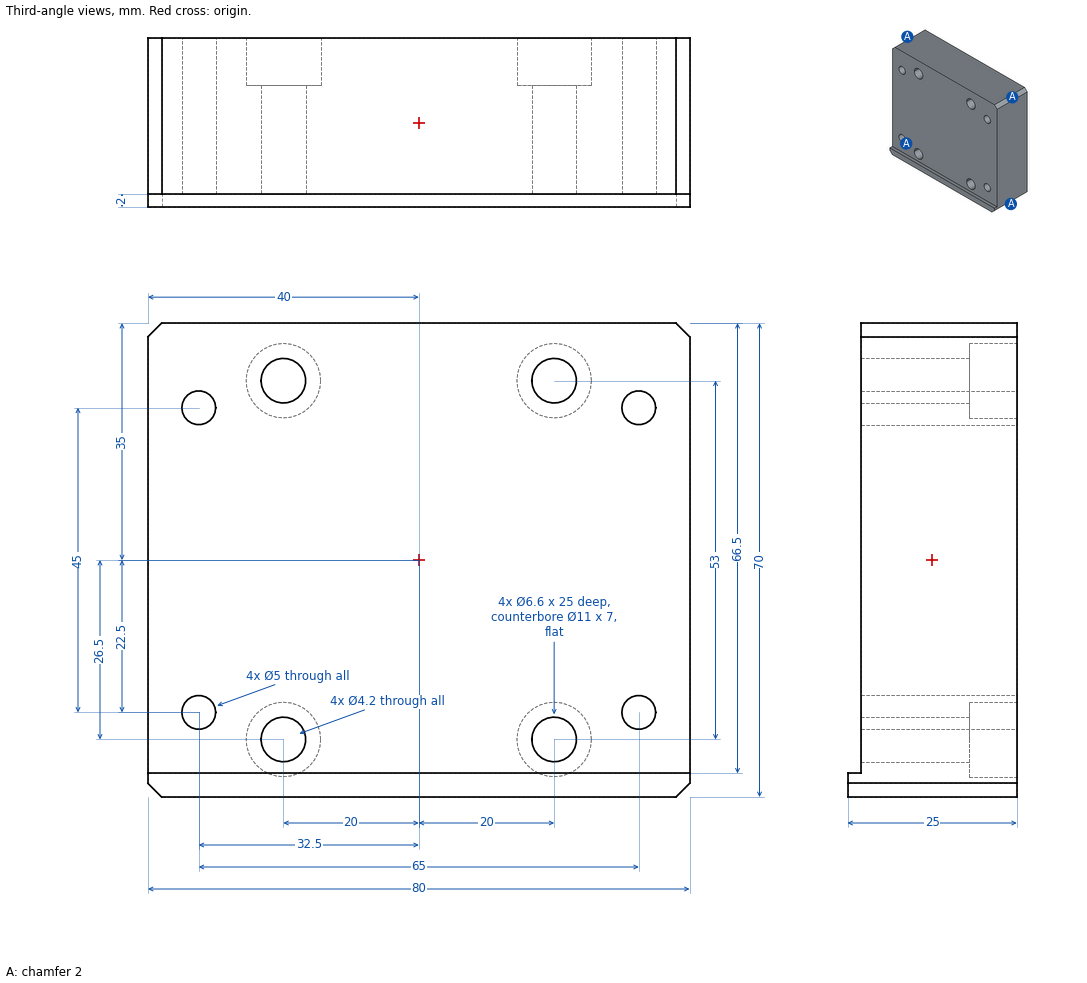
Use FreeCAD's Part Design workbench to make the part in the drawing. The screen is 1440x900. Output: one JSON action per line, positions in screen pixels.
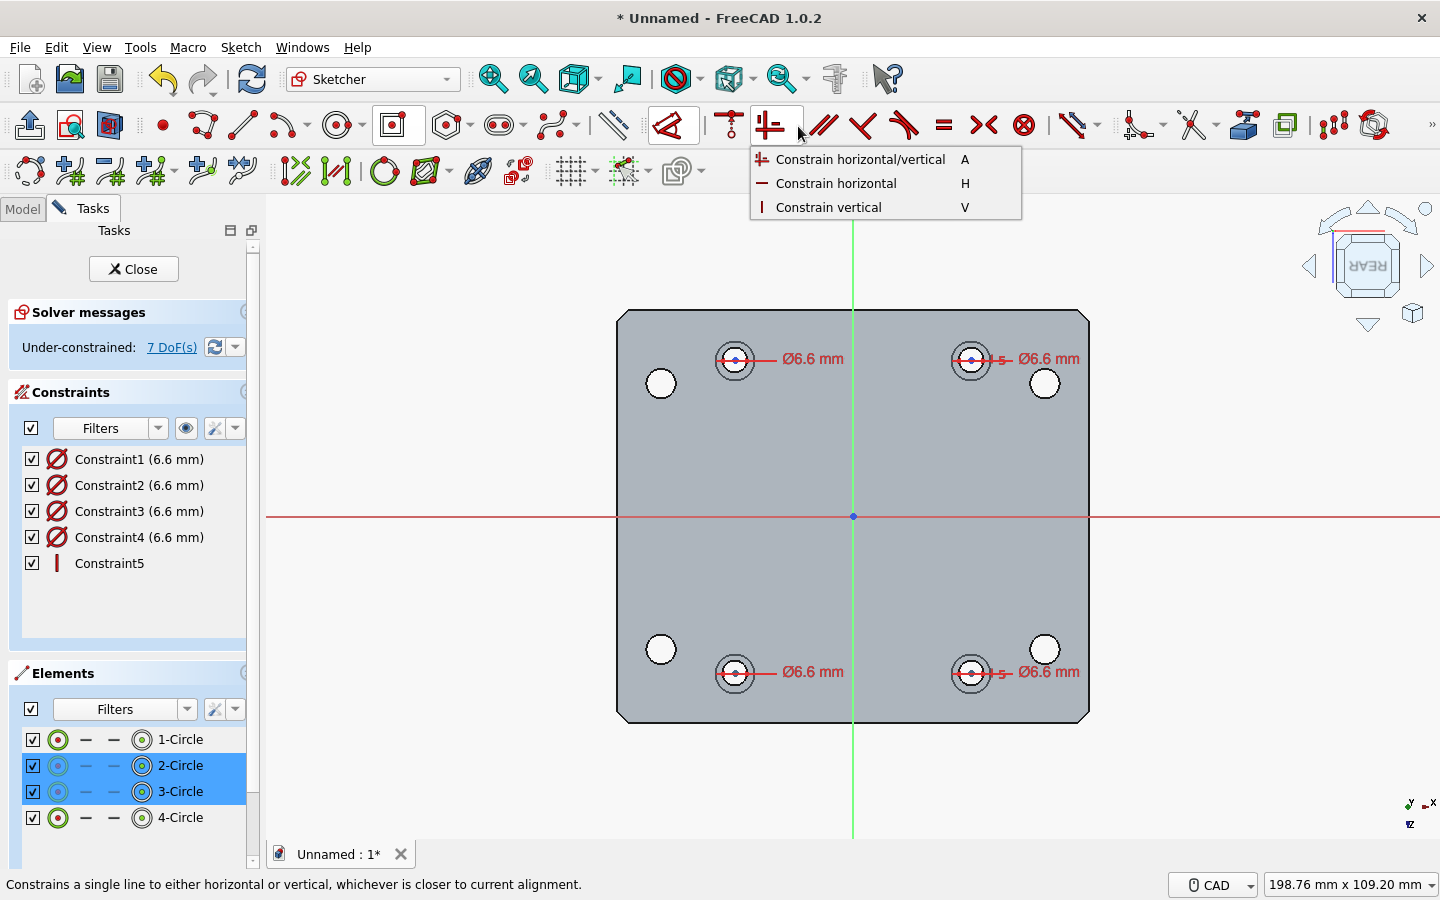
{"action": "left_click", "coordinate": [886, 183]}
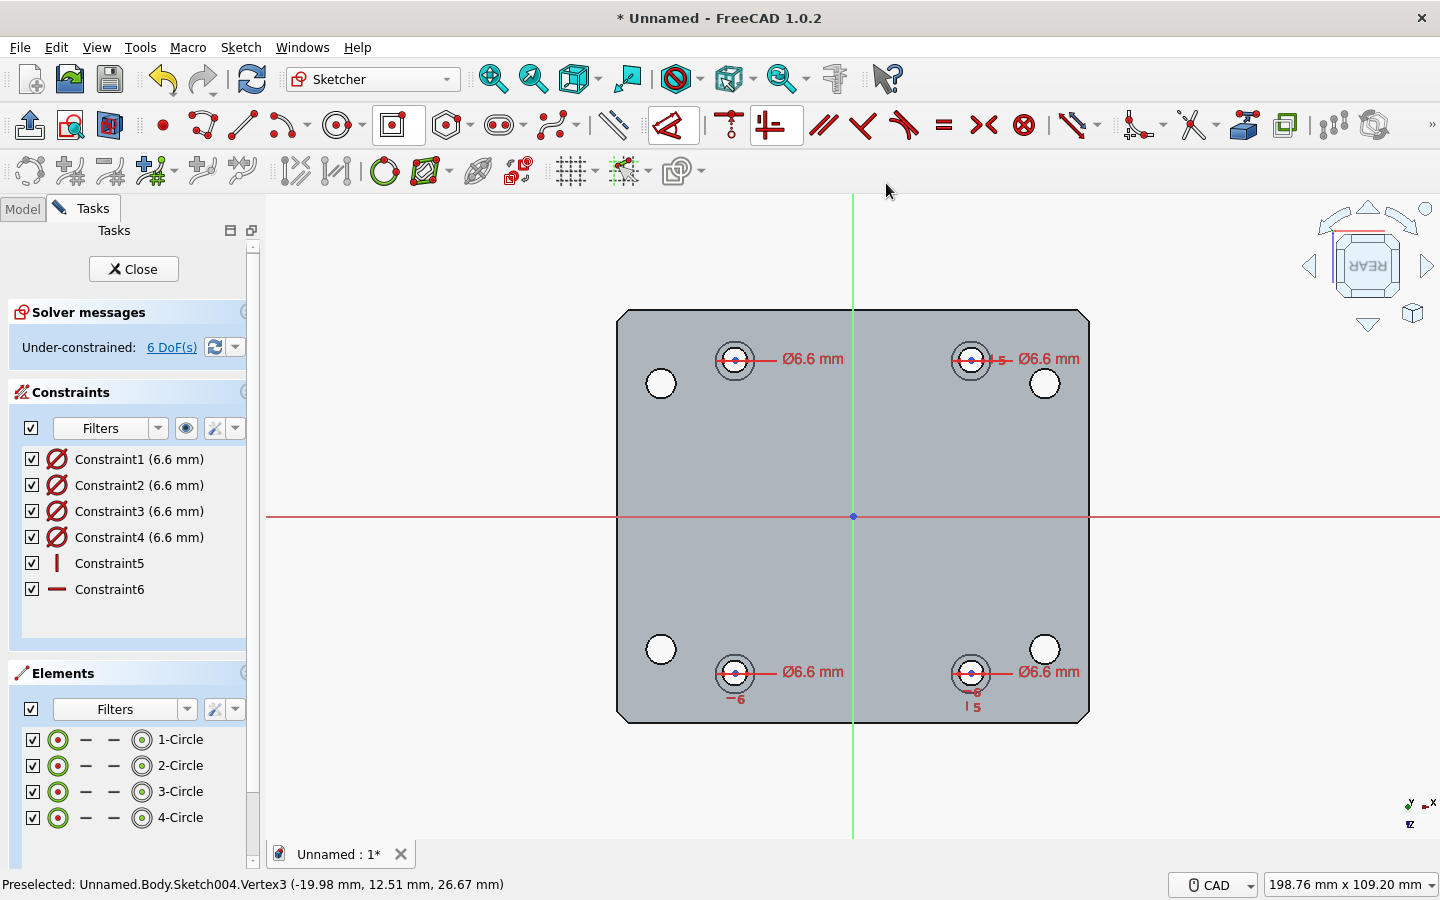
{"action": "left_click", "coordinate": [735, 674]}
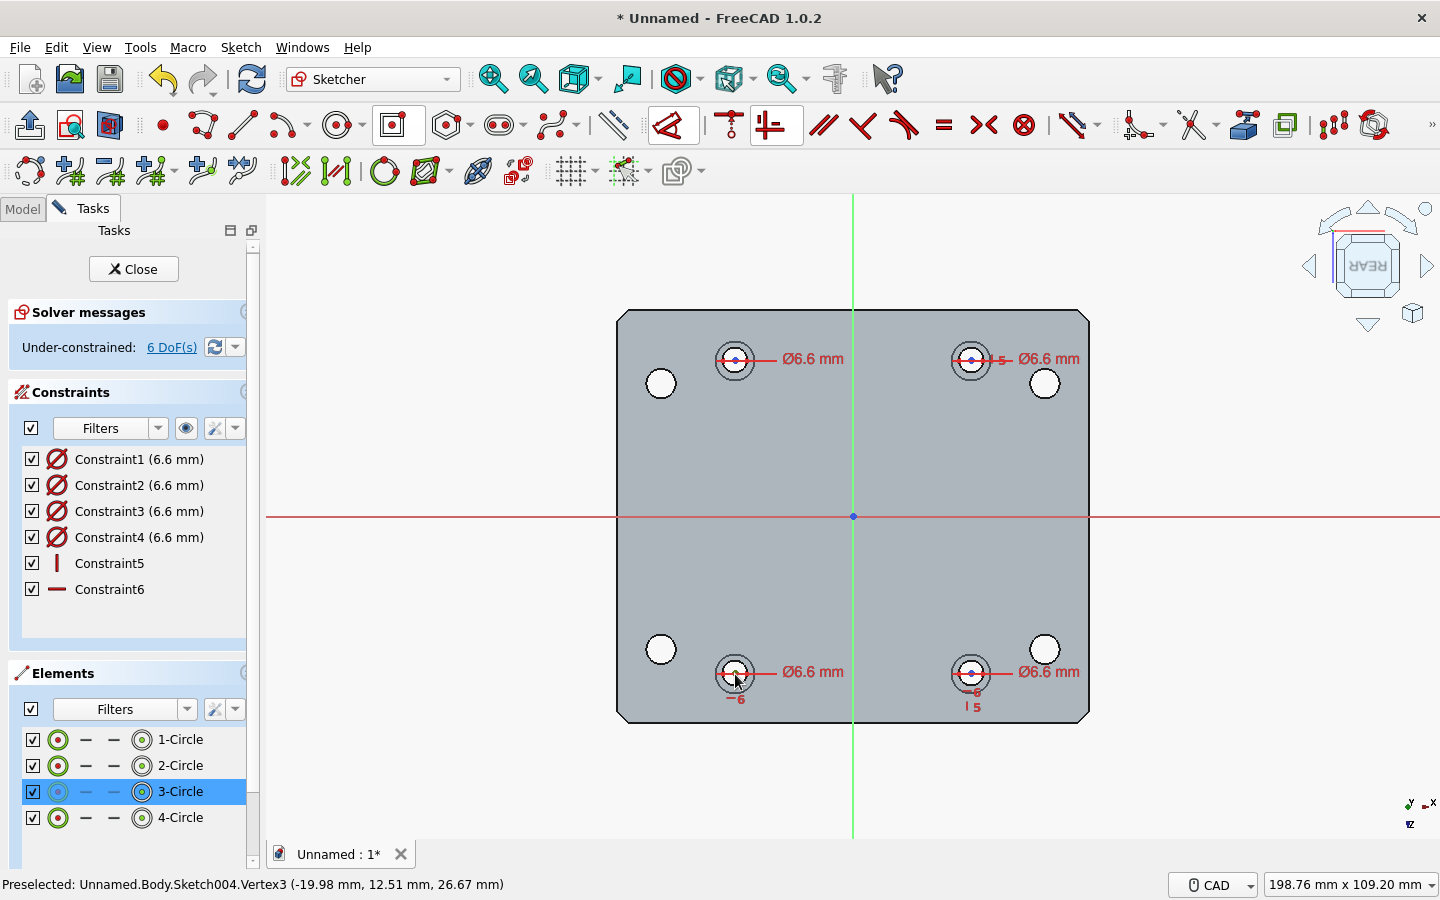
{"action": "left_click", "coordinate": [735, 361]}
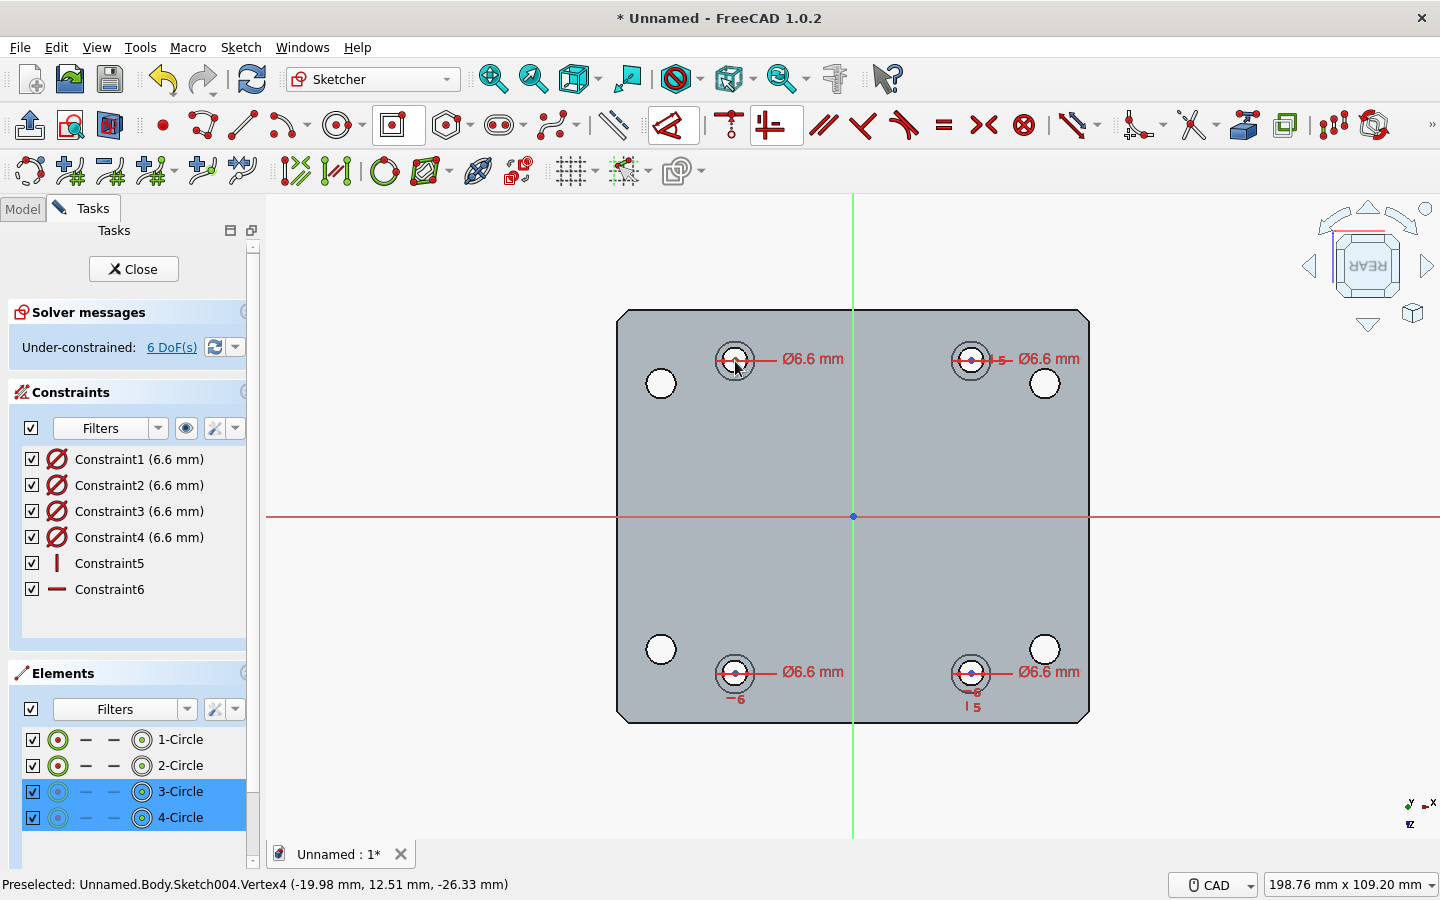
{"action": "left_click", "coordinate": [798, 126]}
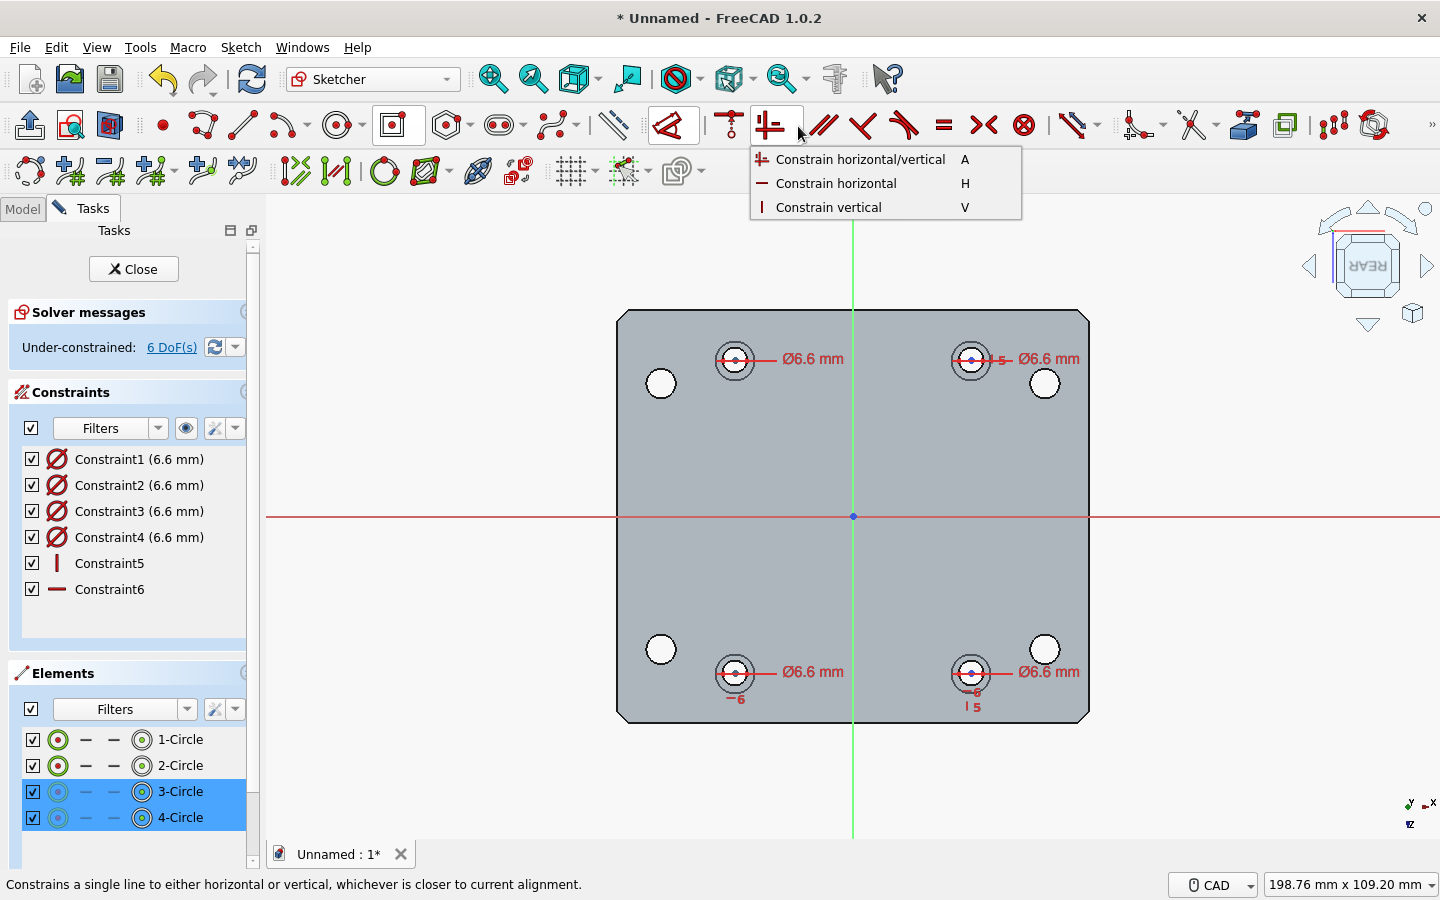
{"action": "left_click", "coordinate": [886, 207]}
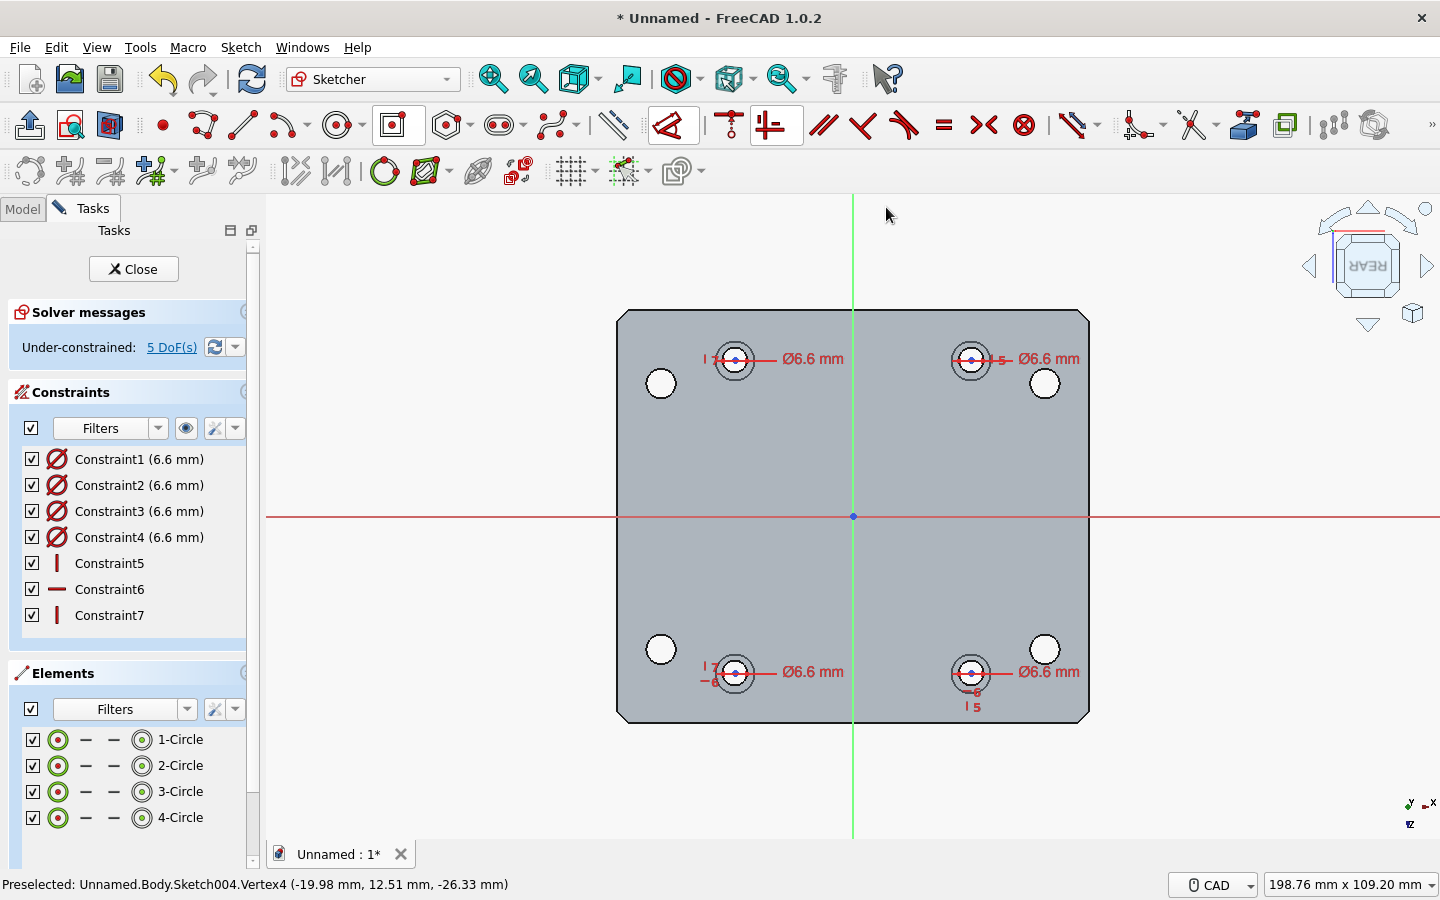
{"action": "left_click", "coordinate": [971, 361]}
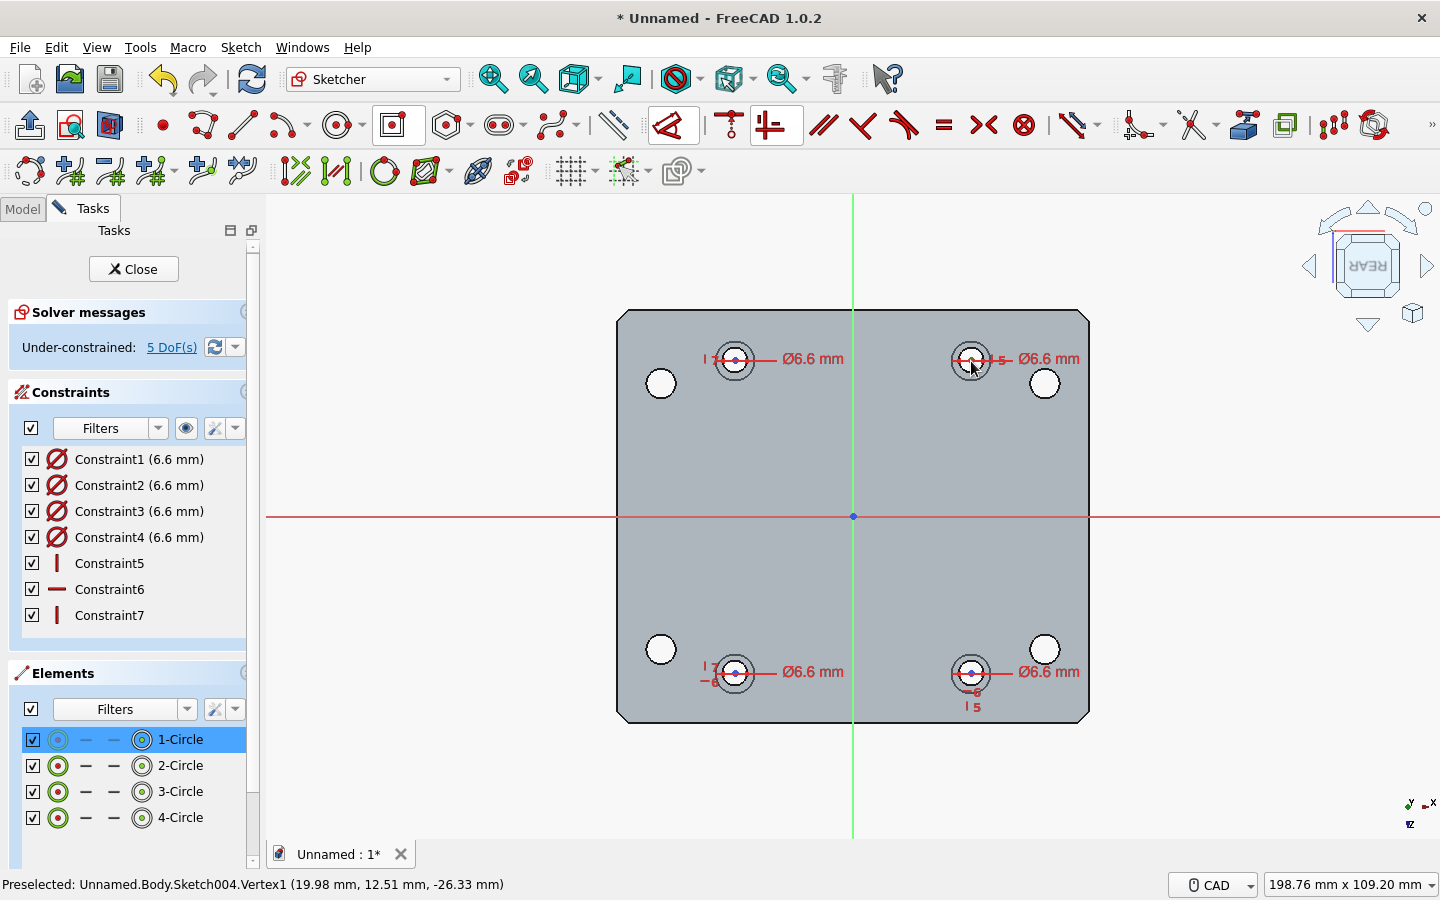
{"action": "left_click", "coordinate": [735, 361]}